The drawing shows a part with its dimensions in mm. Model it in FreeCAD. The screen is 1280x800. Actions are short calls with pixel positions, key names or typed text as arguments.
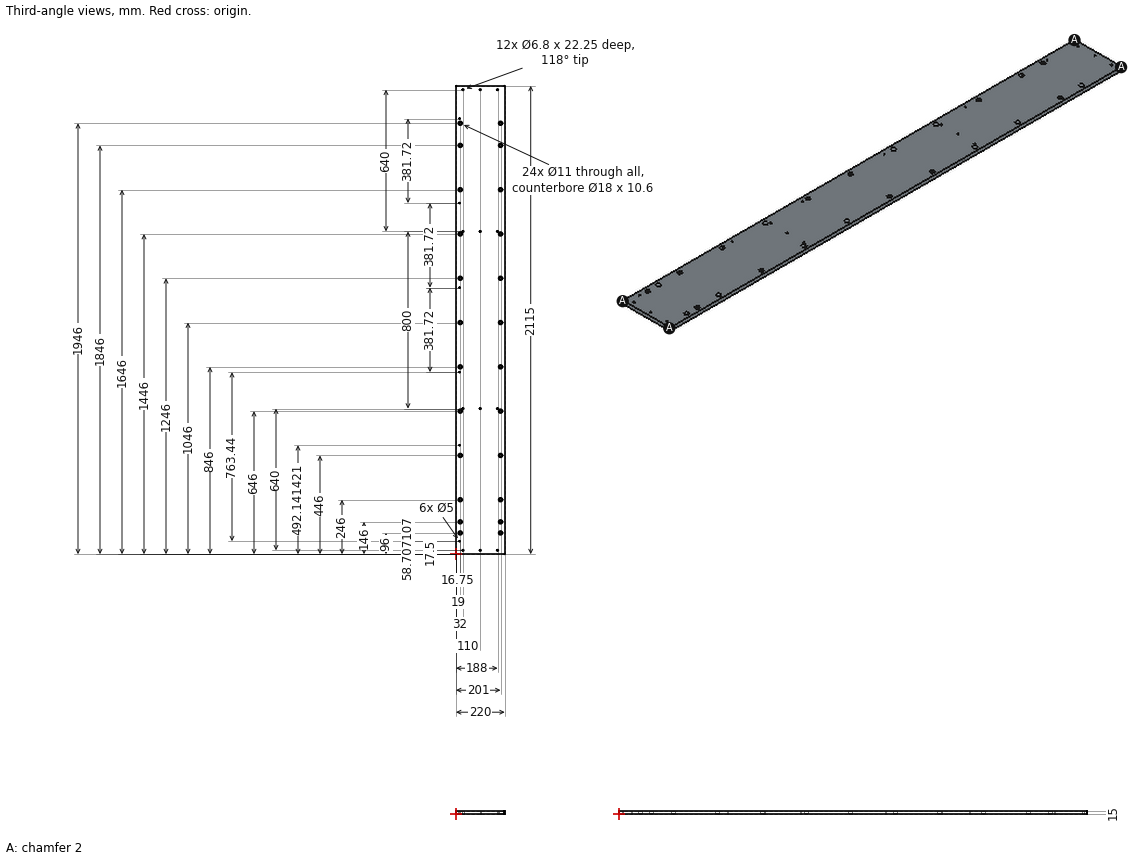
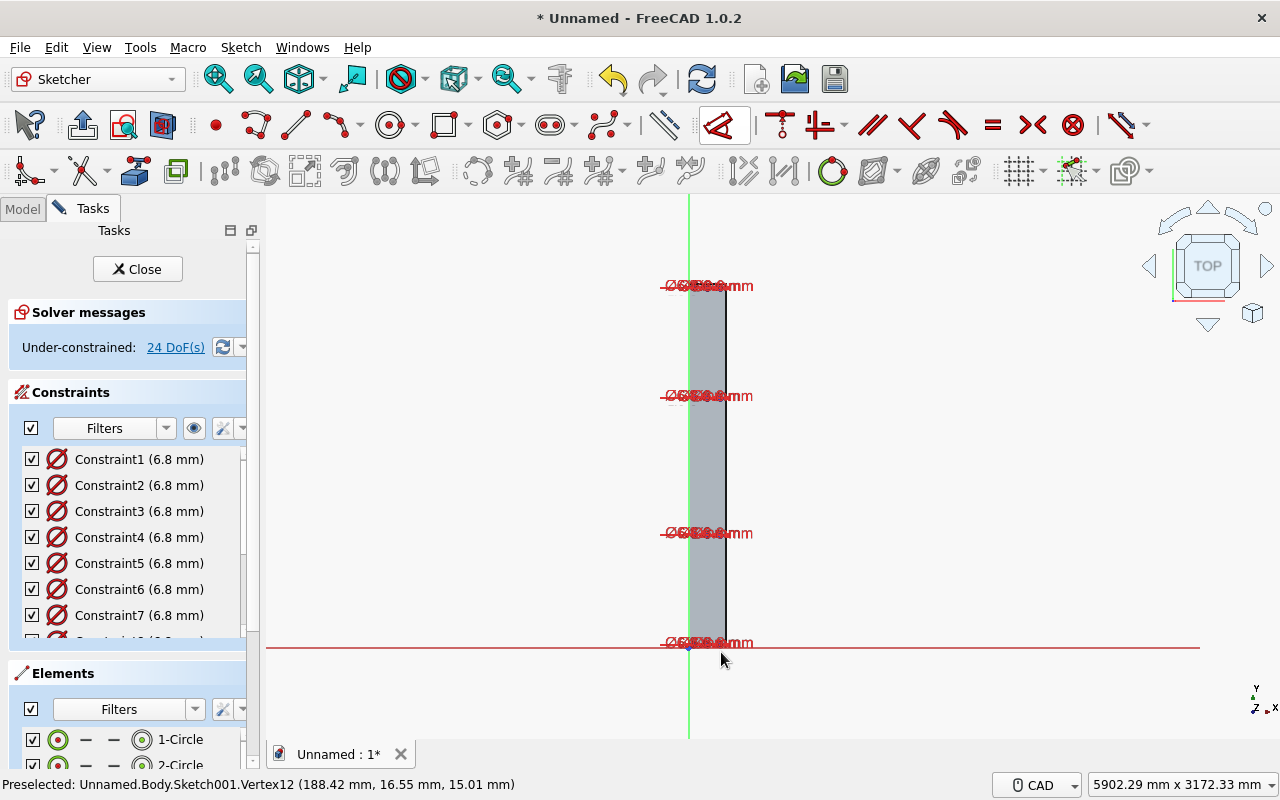
click(694, 288)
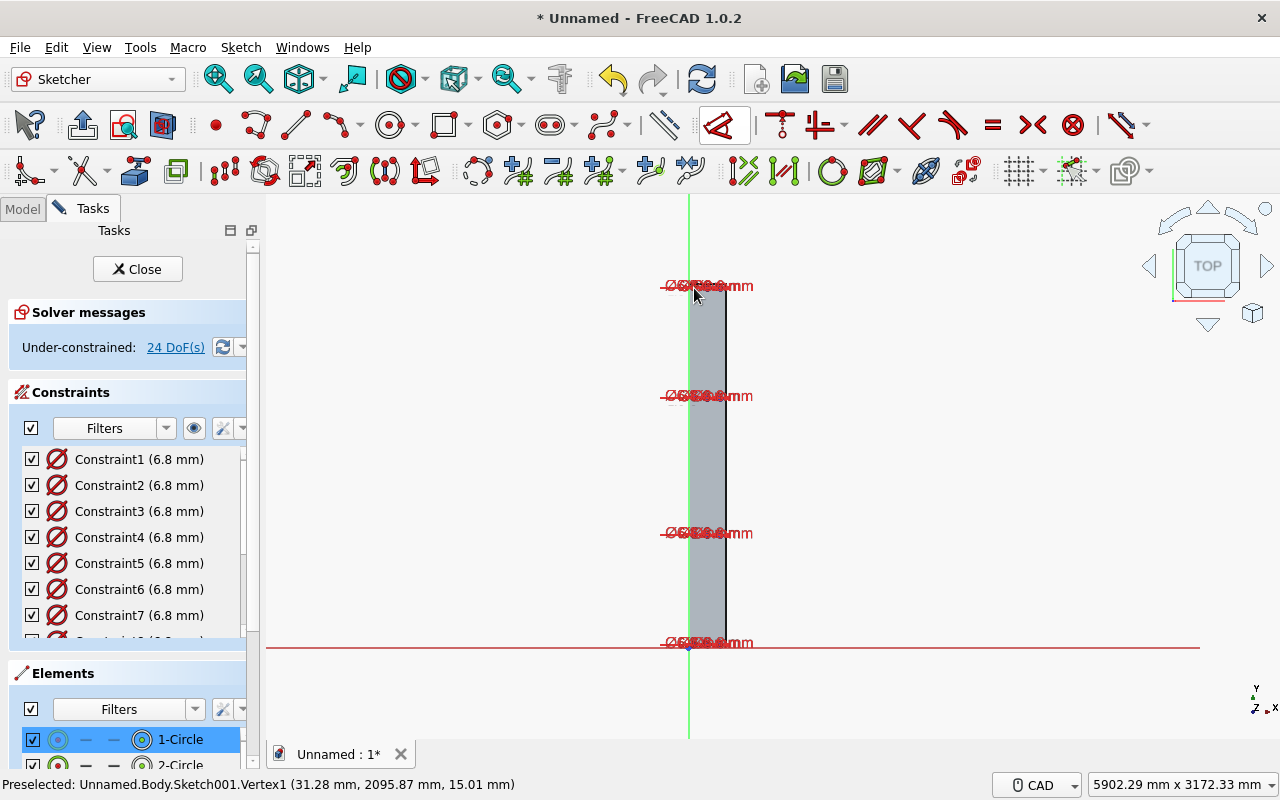
click(694, 398)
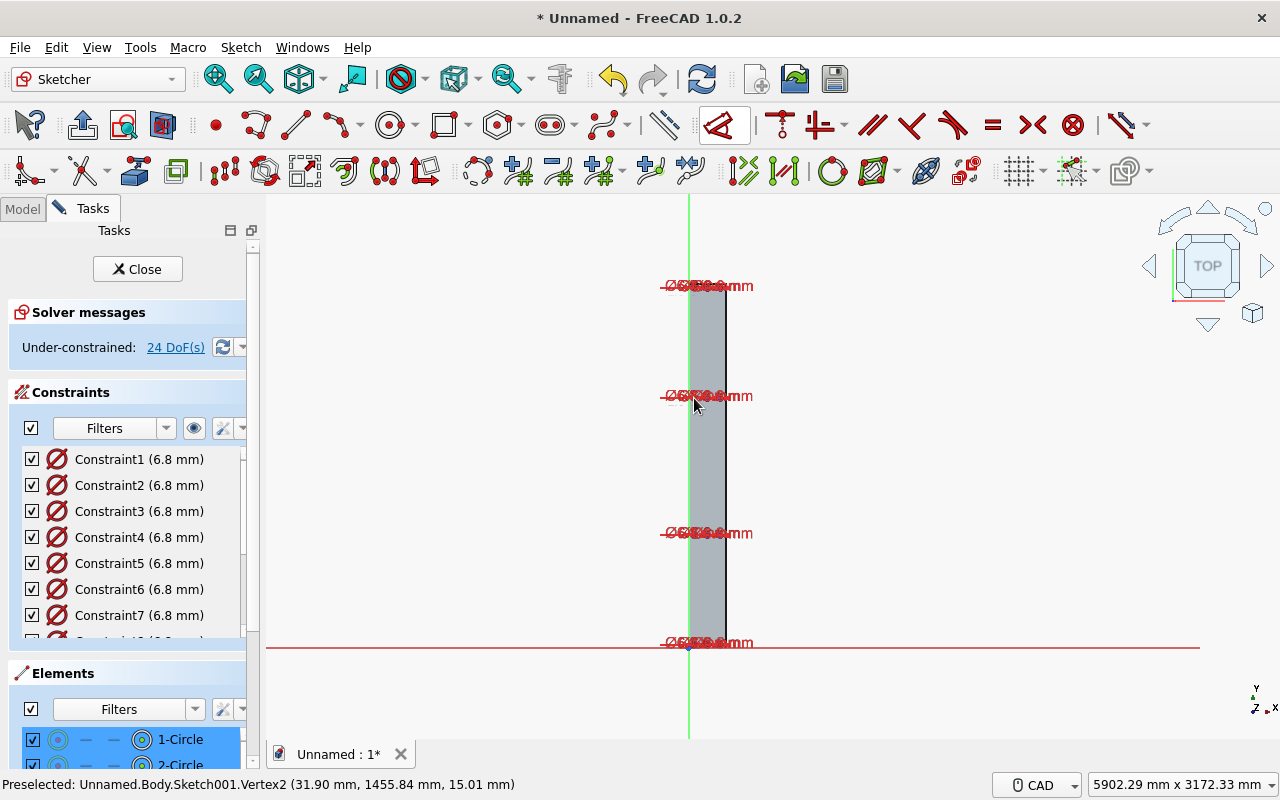
click(846, 126)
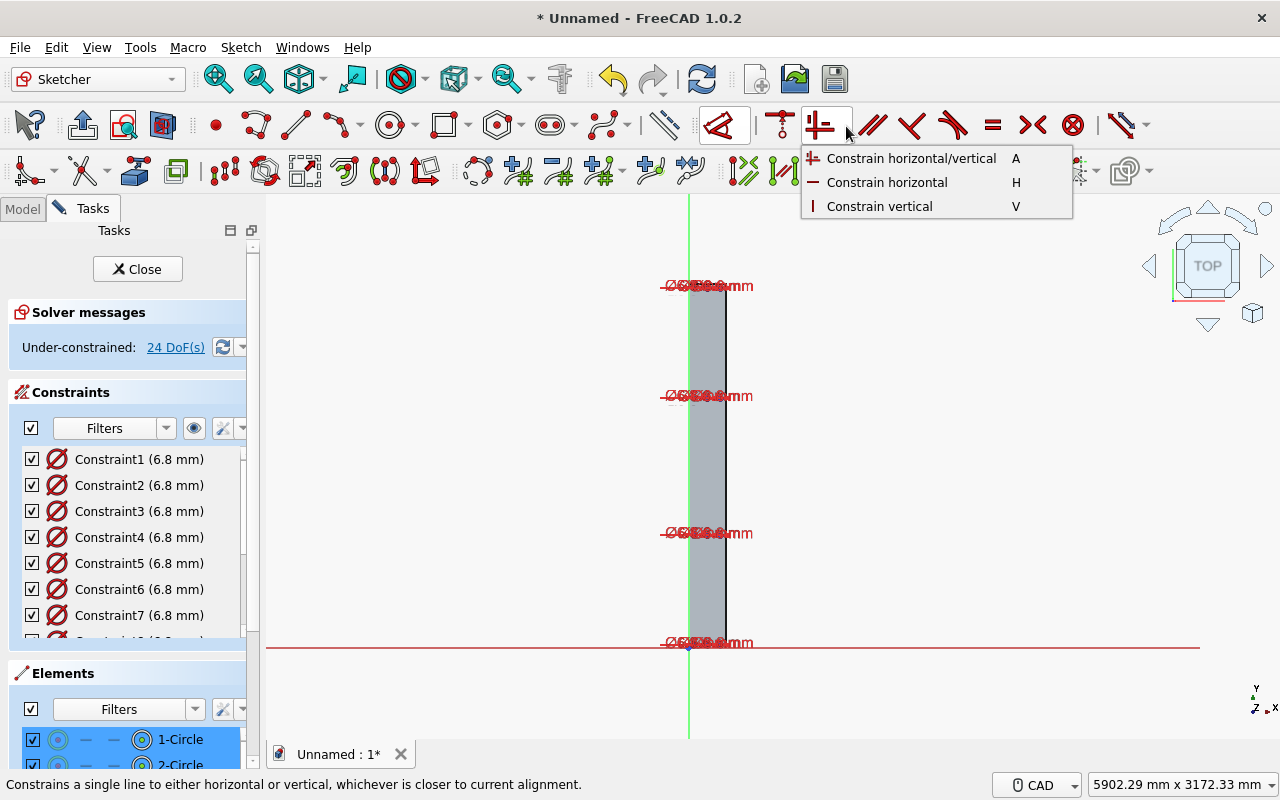
click(937, 206)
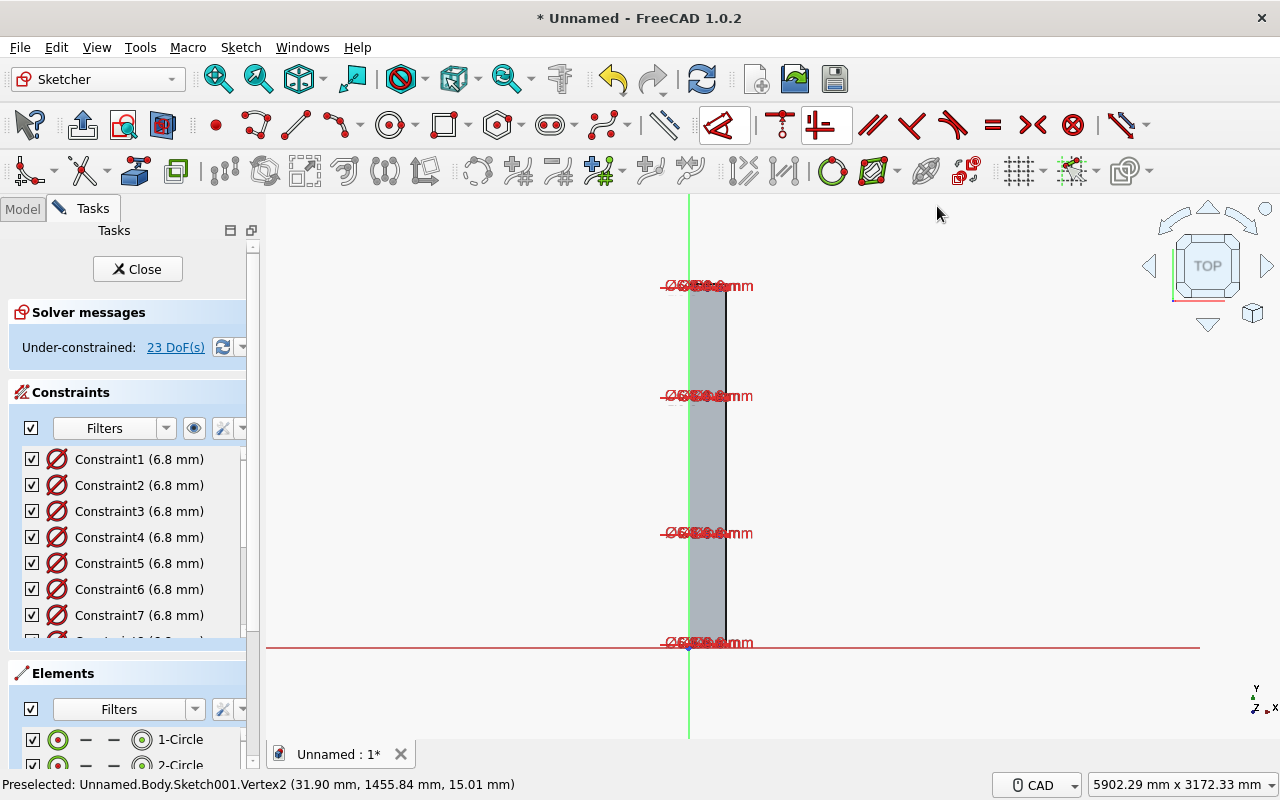
click(694, 398)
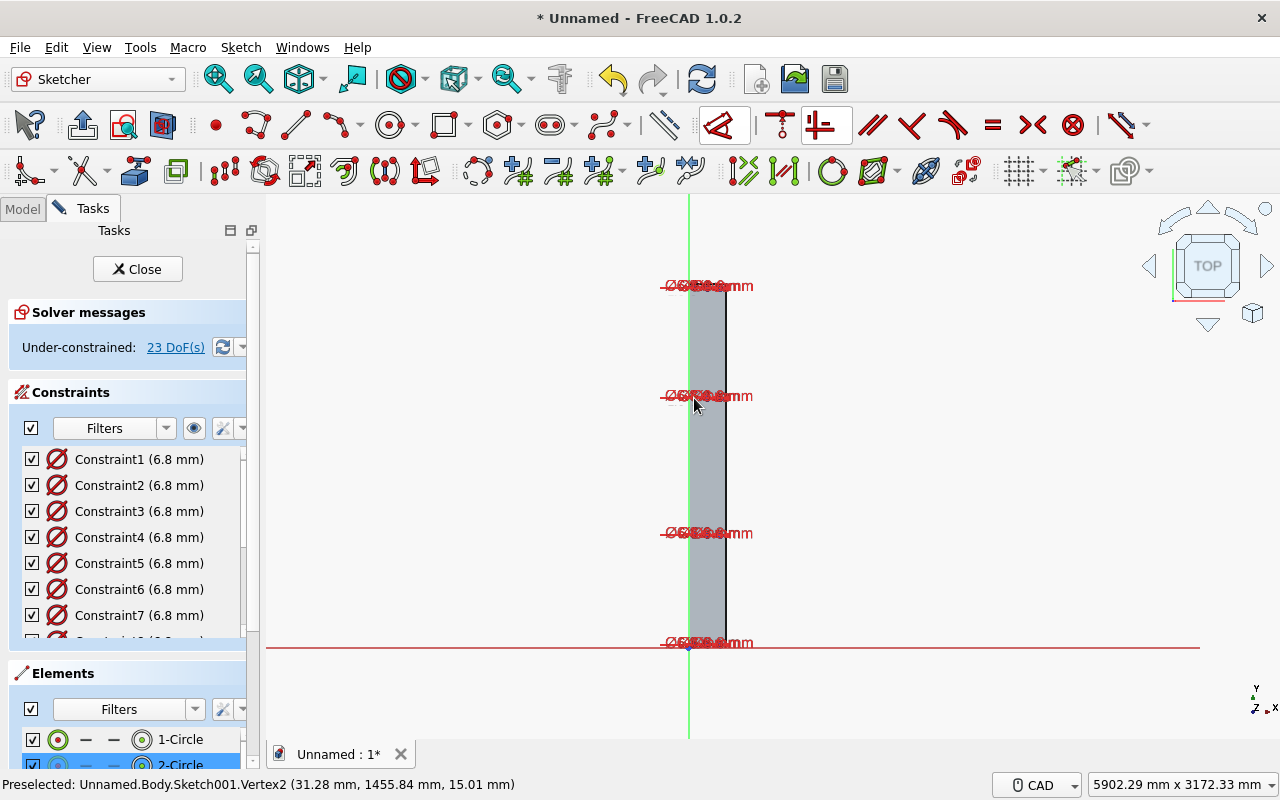
click(694, 535)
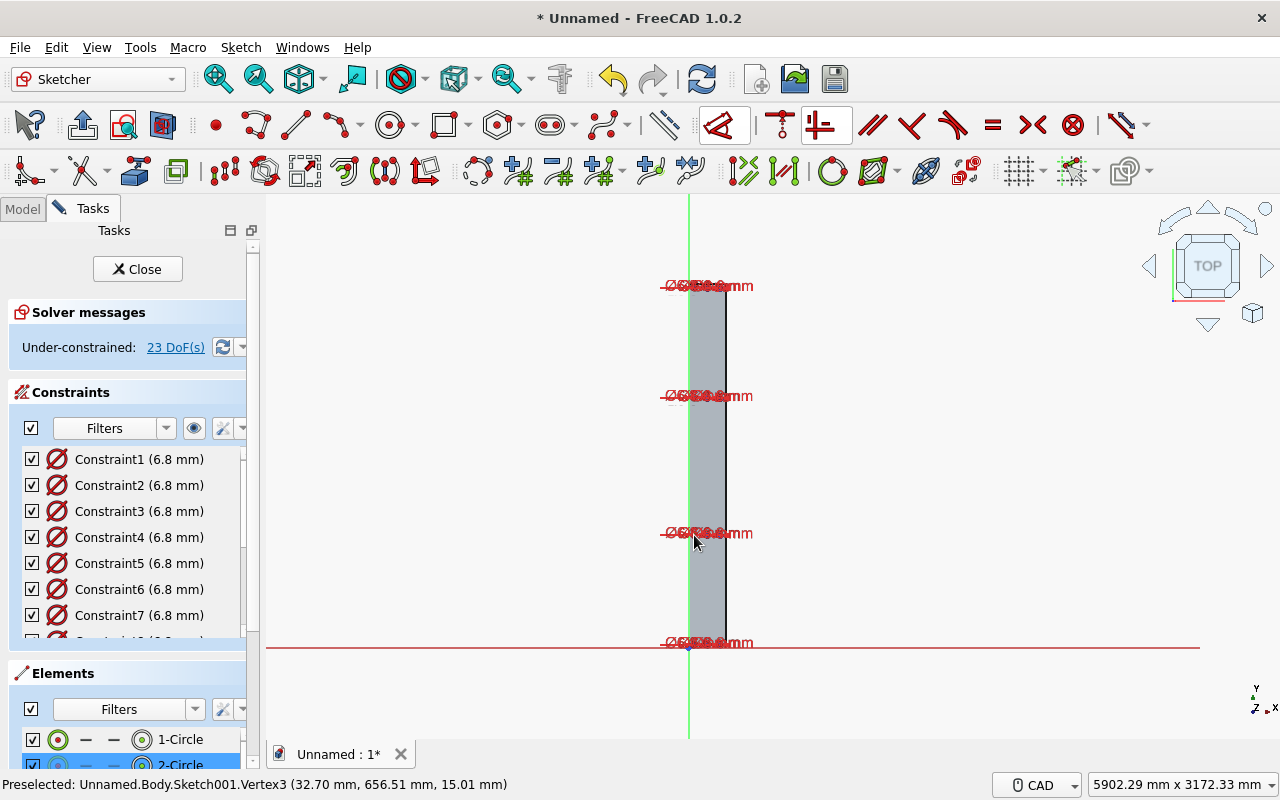
click(846, 126)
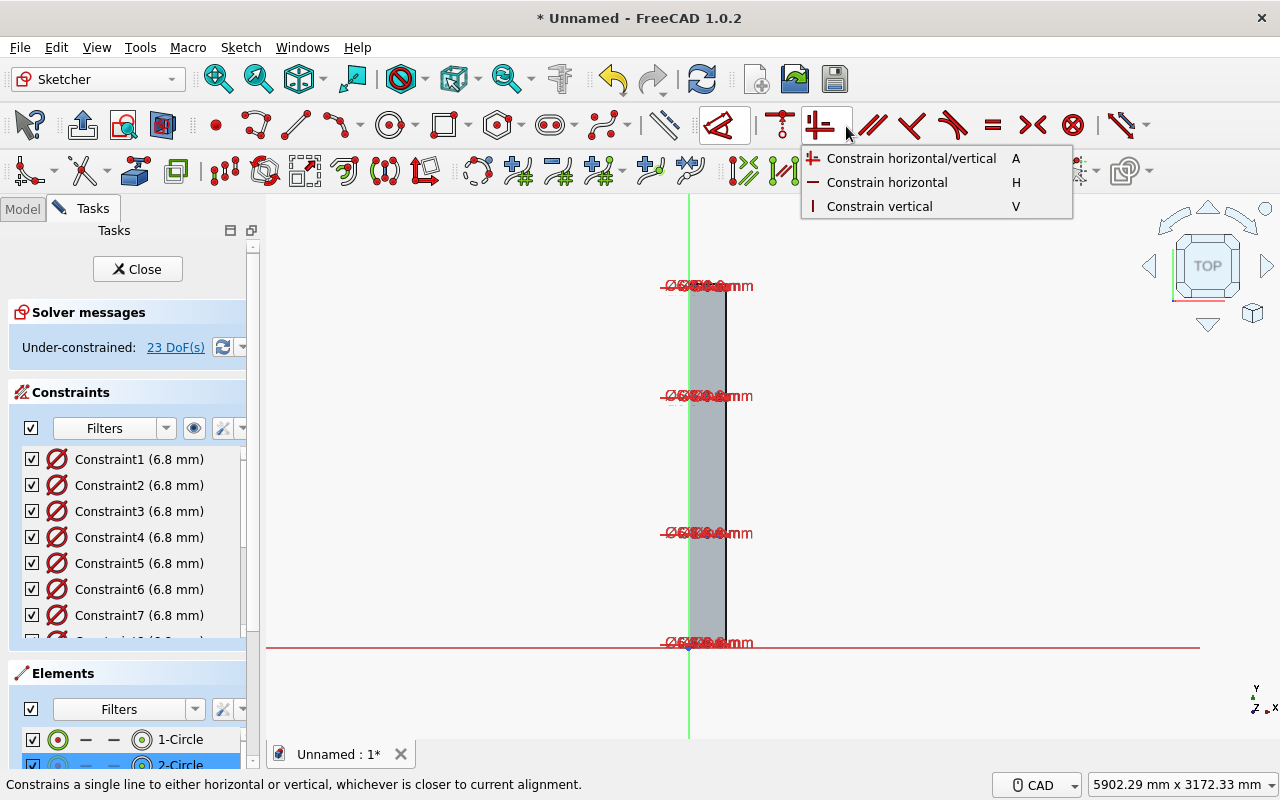
click(937, 206)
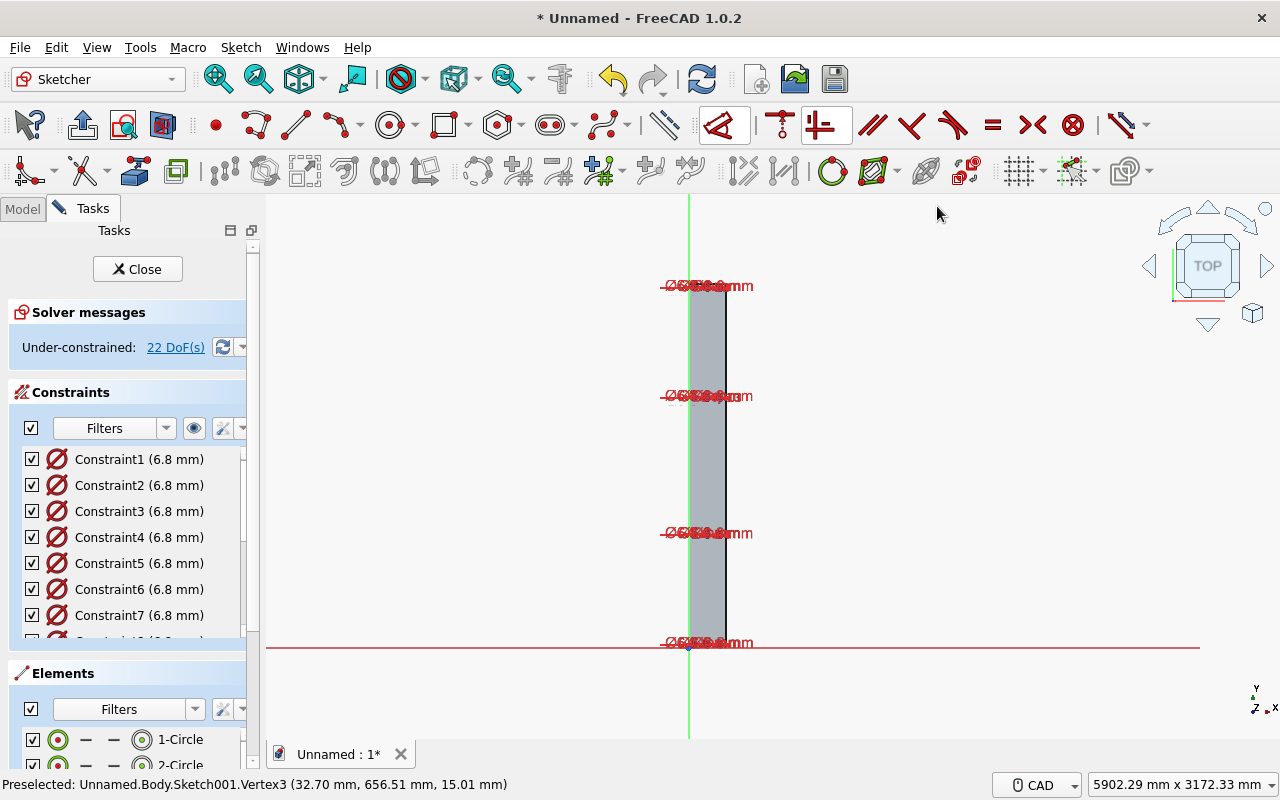
click(694, 535)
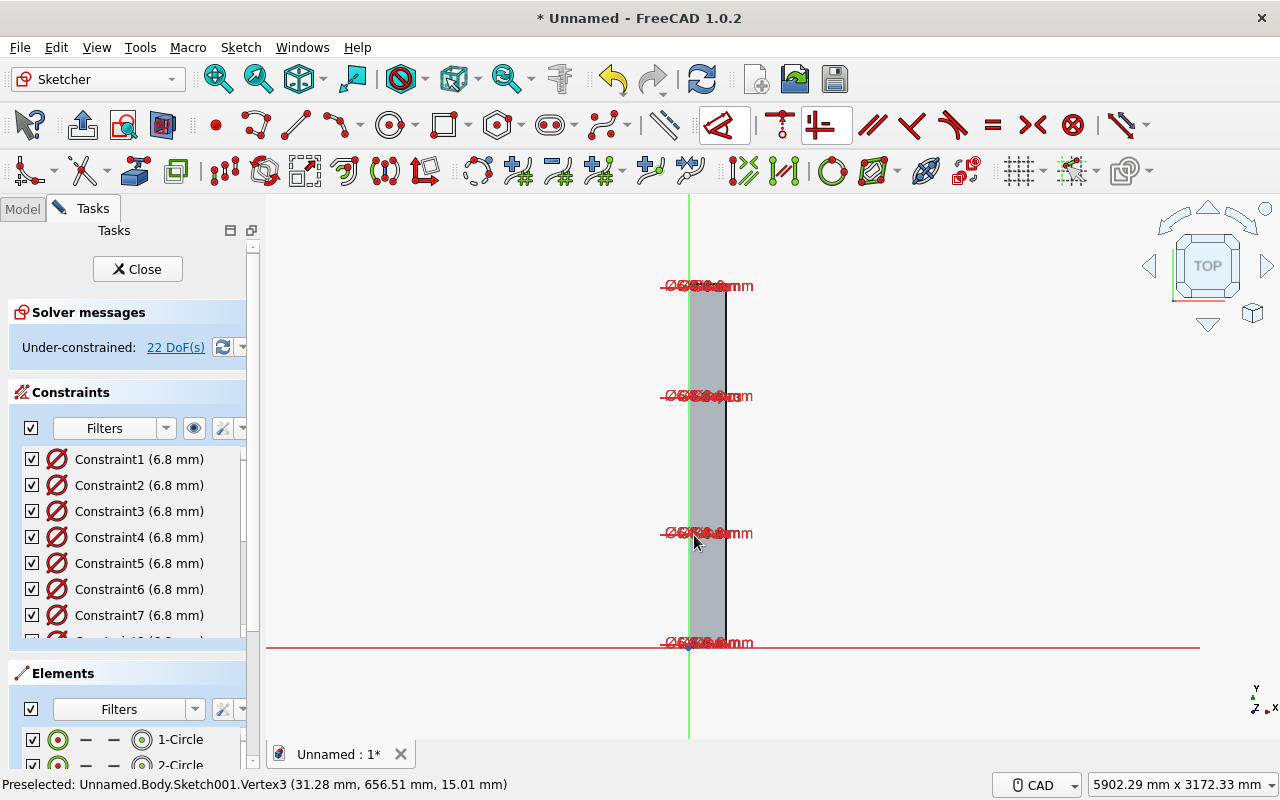
scroll(694, 645, up, 4)